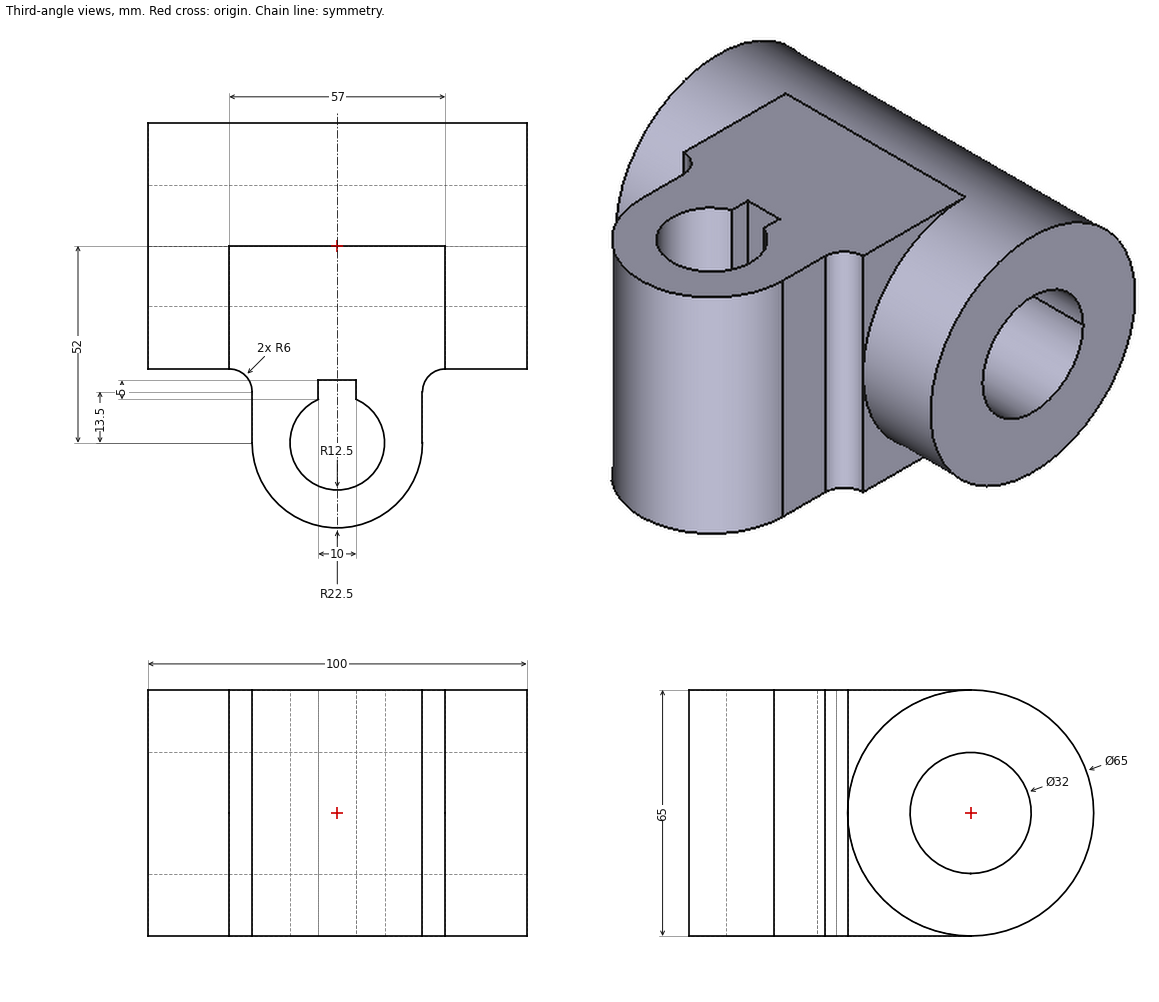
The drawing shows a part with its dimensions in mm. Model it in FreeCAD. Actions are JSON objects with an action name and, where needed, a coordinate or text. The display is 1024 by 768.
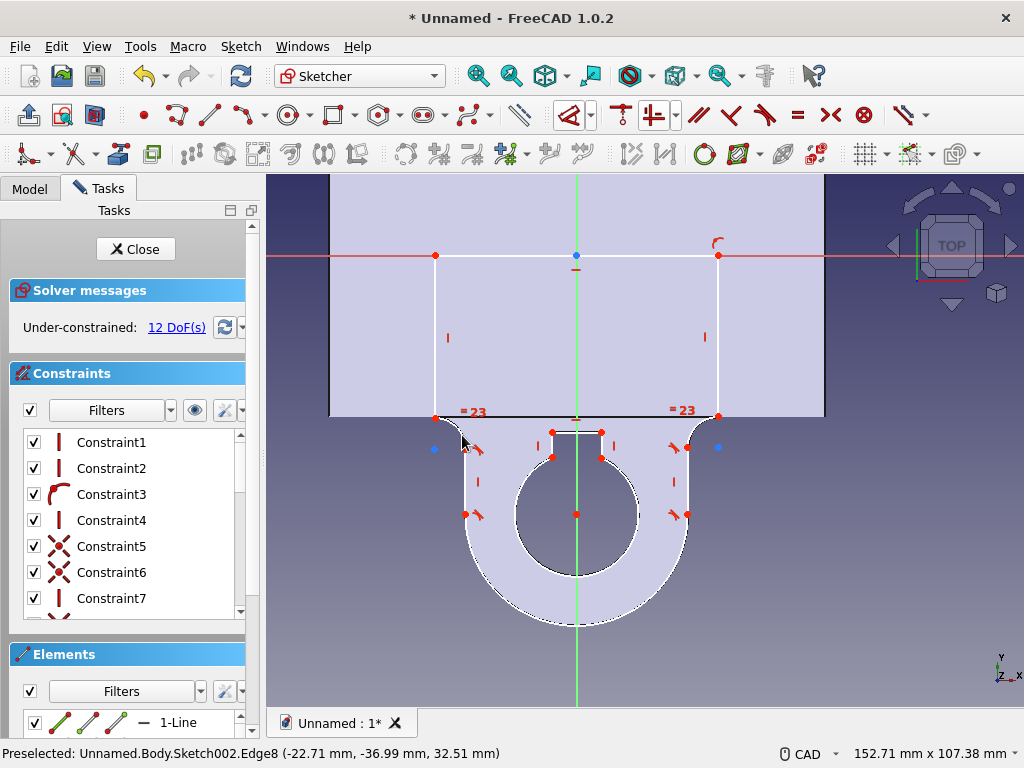
{"action": "left_click", "coordinate": [576, 515]}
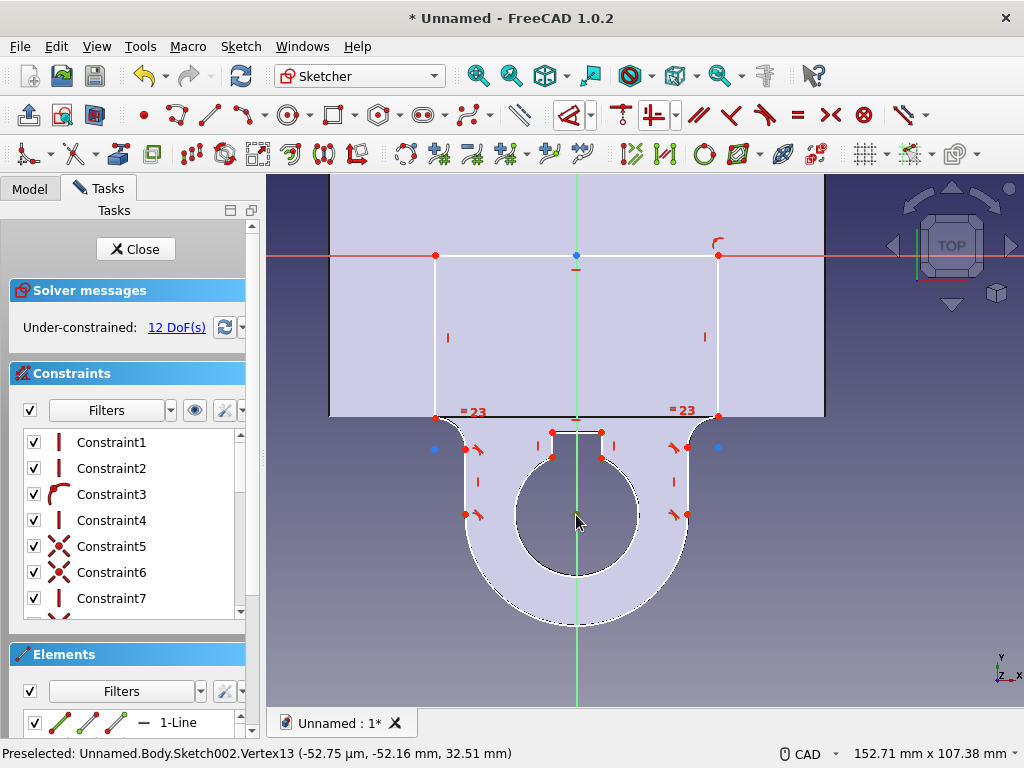
{"action": "left_click", "coordinate": [577, 543]}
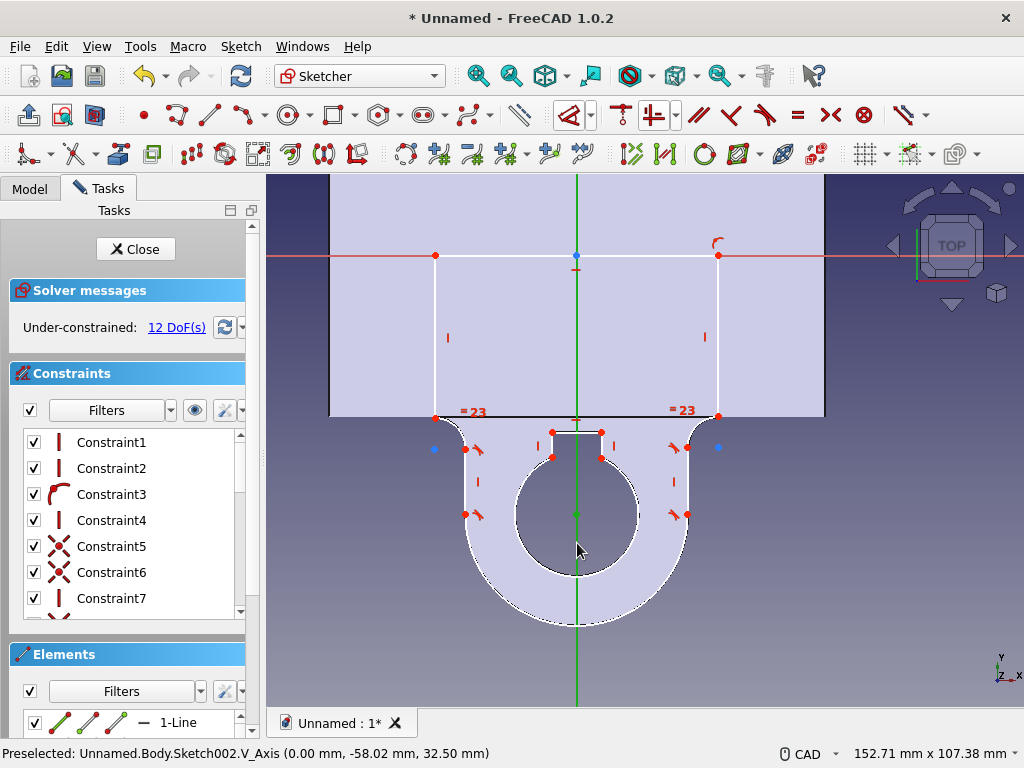
{"action": "key", "text": "c"}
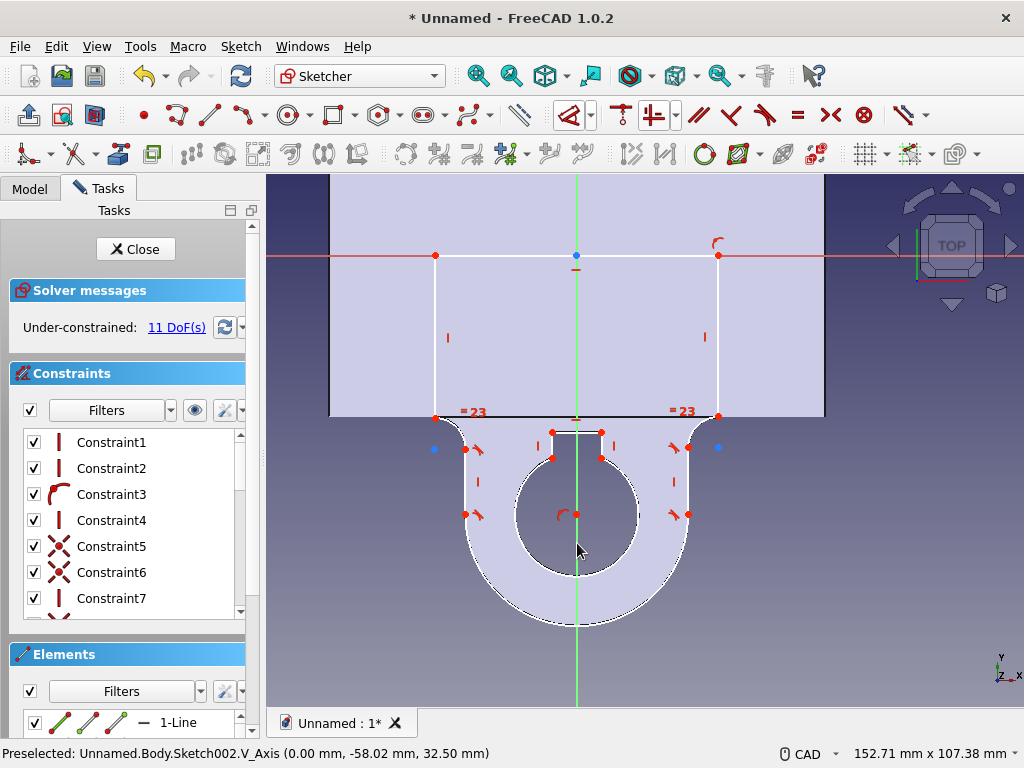
{"action": "left_click", "coordinate": [718, 417]}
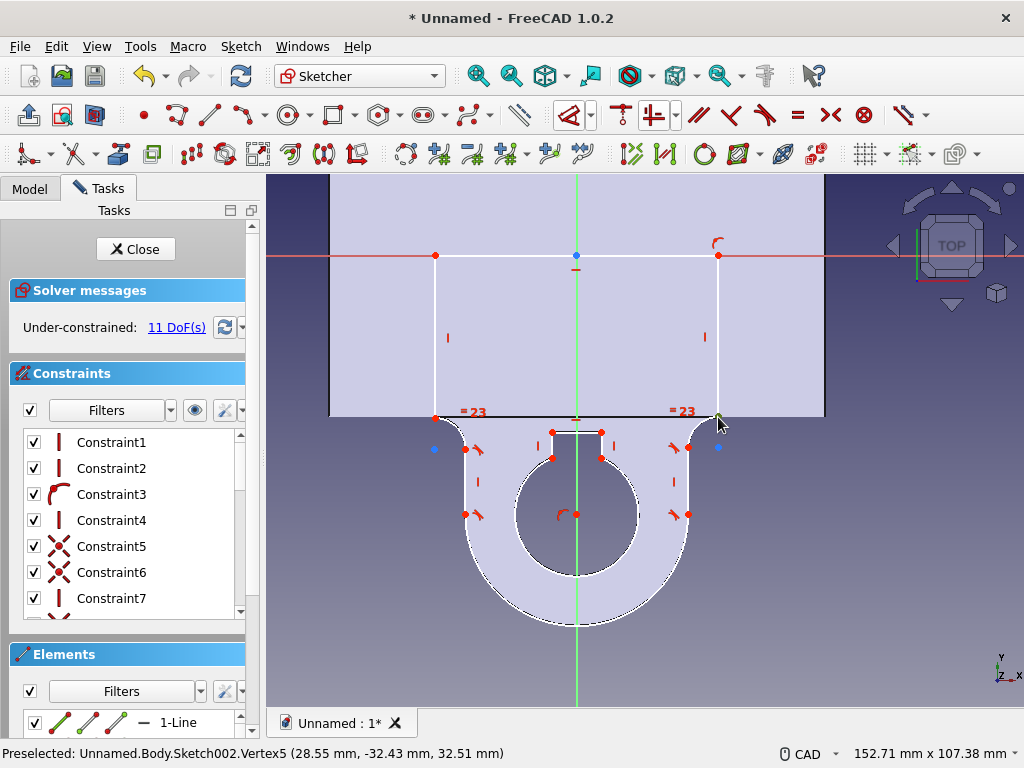
{"action": "left_click", "coordinate": [435, 418]}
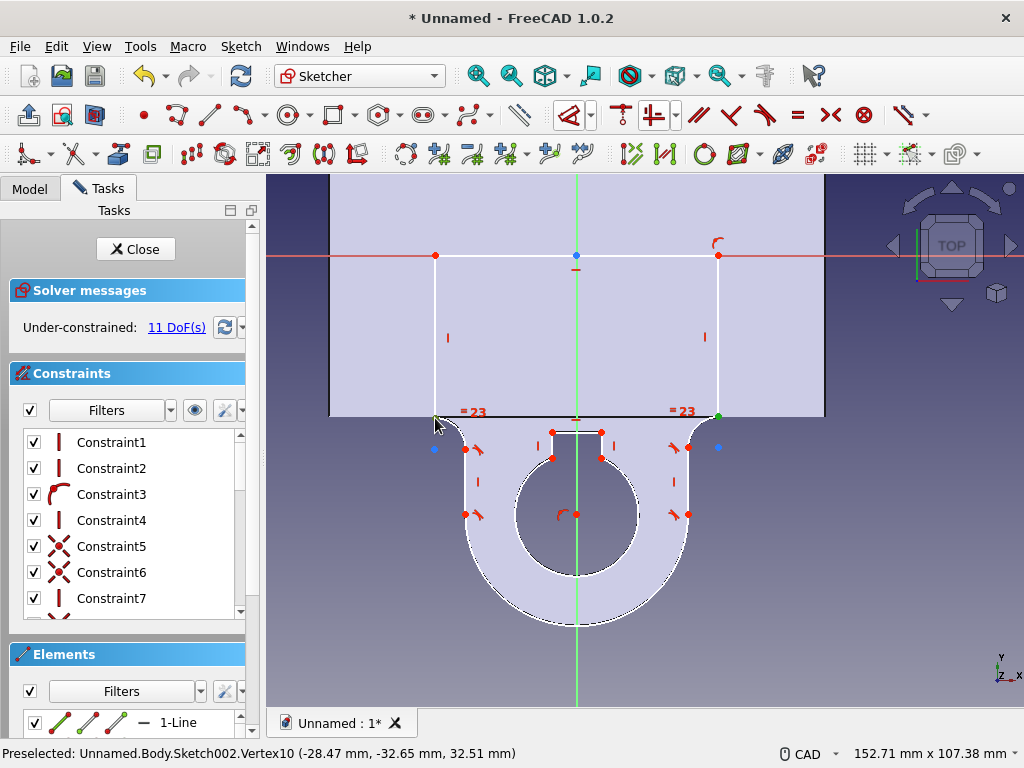
{"action": "left_click", "coordinate": [577, 543]}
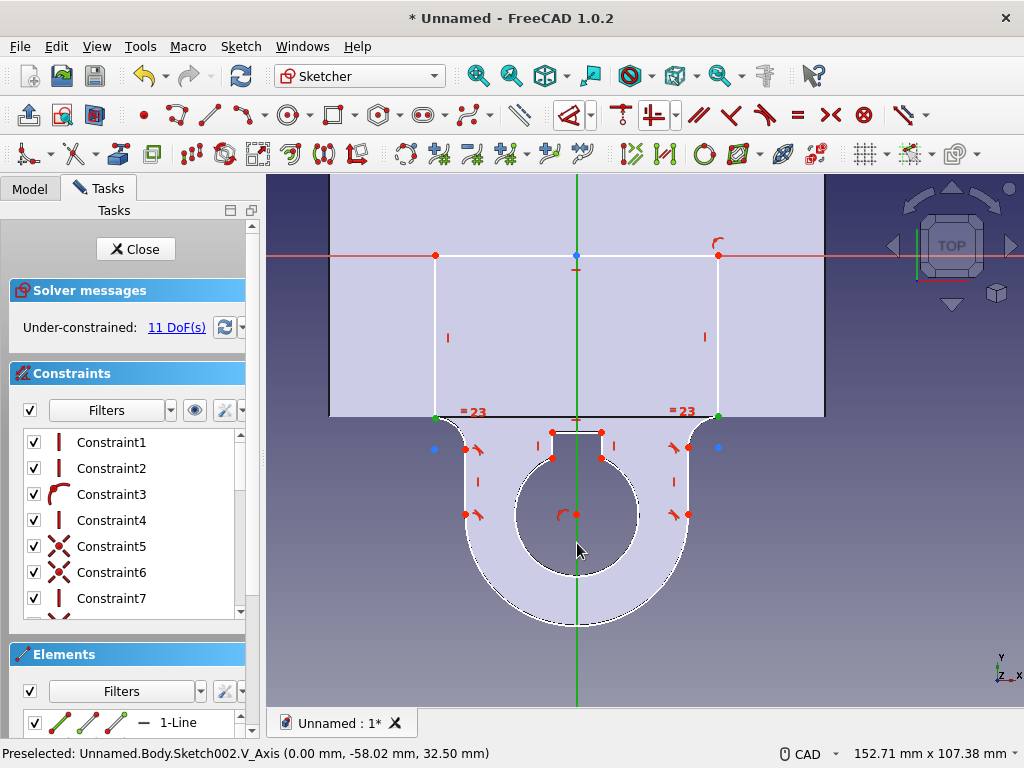
{"action": "left_click", "coordinate": [831, 116]}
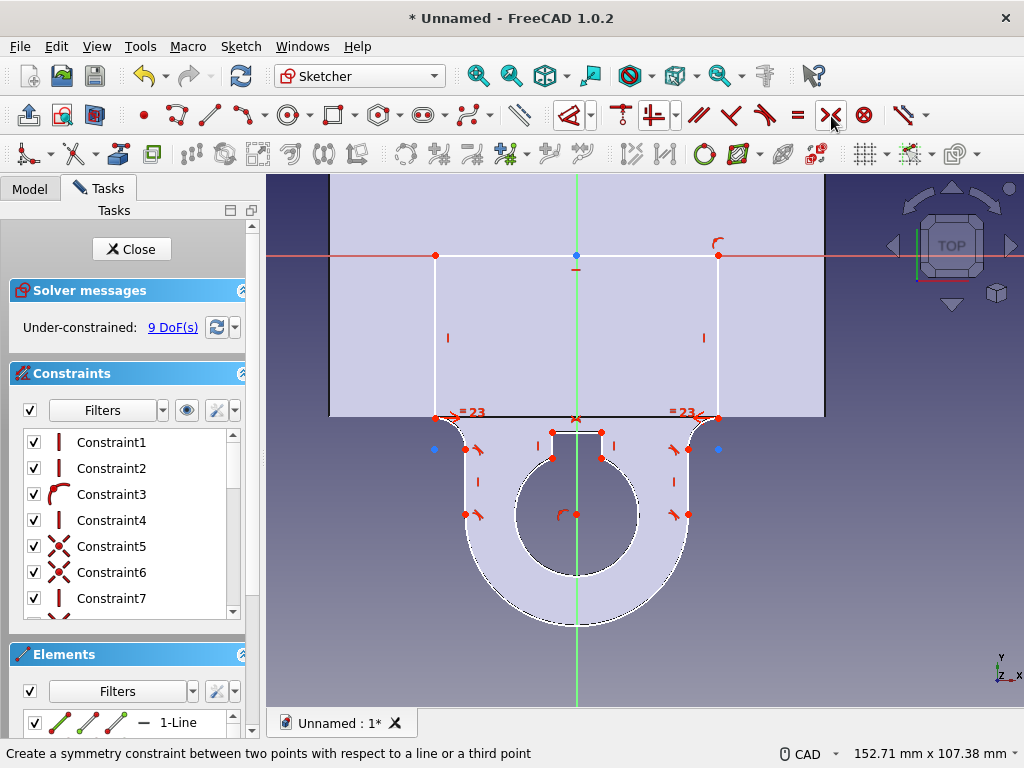
{"action": "left_click", "coordinate": [511, 605]}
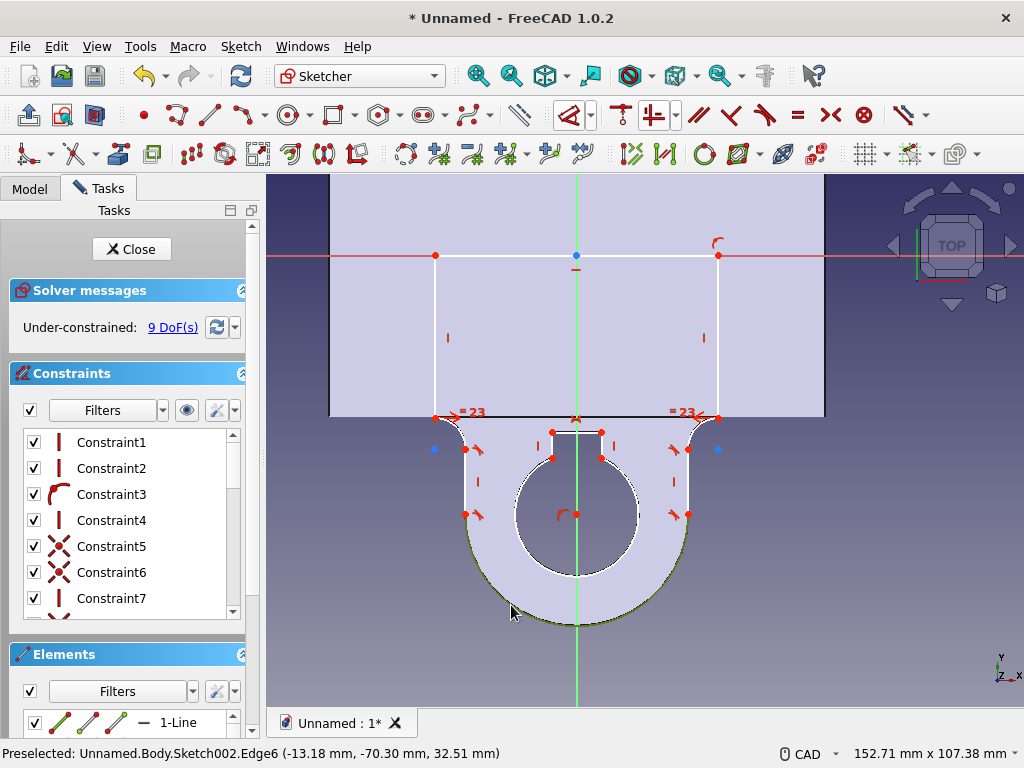
{"action": "key", "text": "k r"}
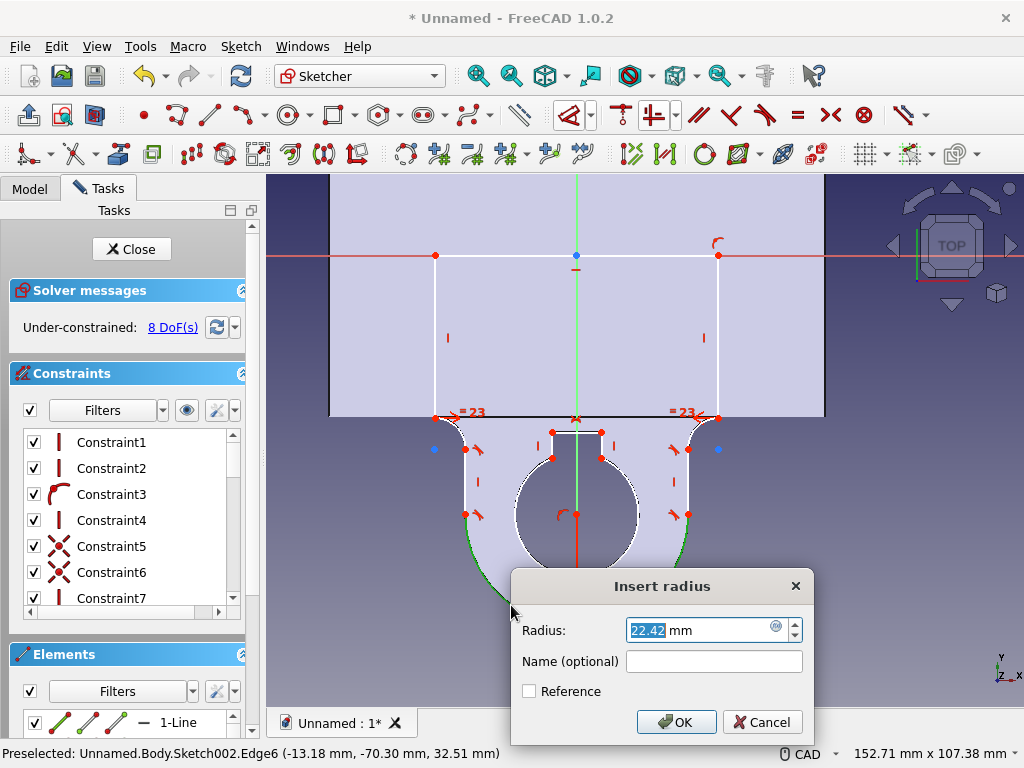
{"action": "type", "text": "22.5"}
{"action": "key", "text": "Return"}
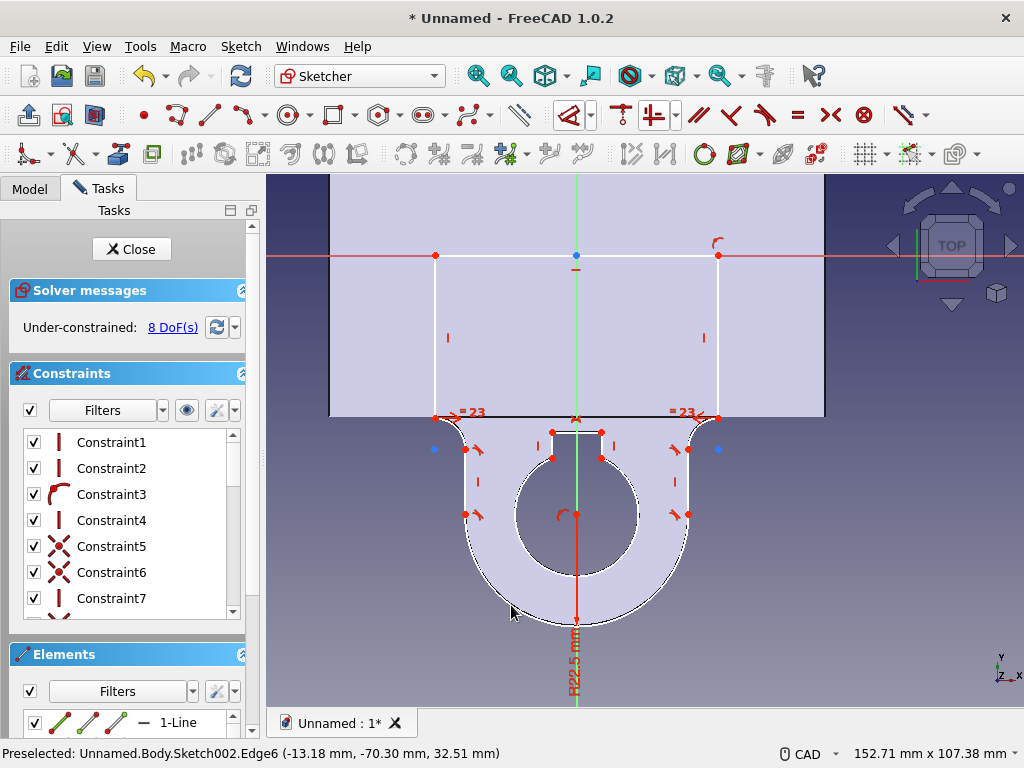
{"action": "scroll", "coordinate": [705, 422], "scroll_direction": "up", "scroll_amount": 2}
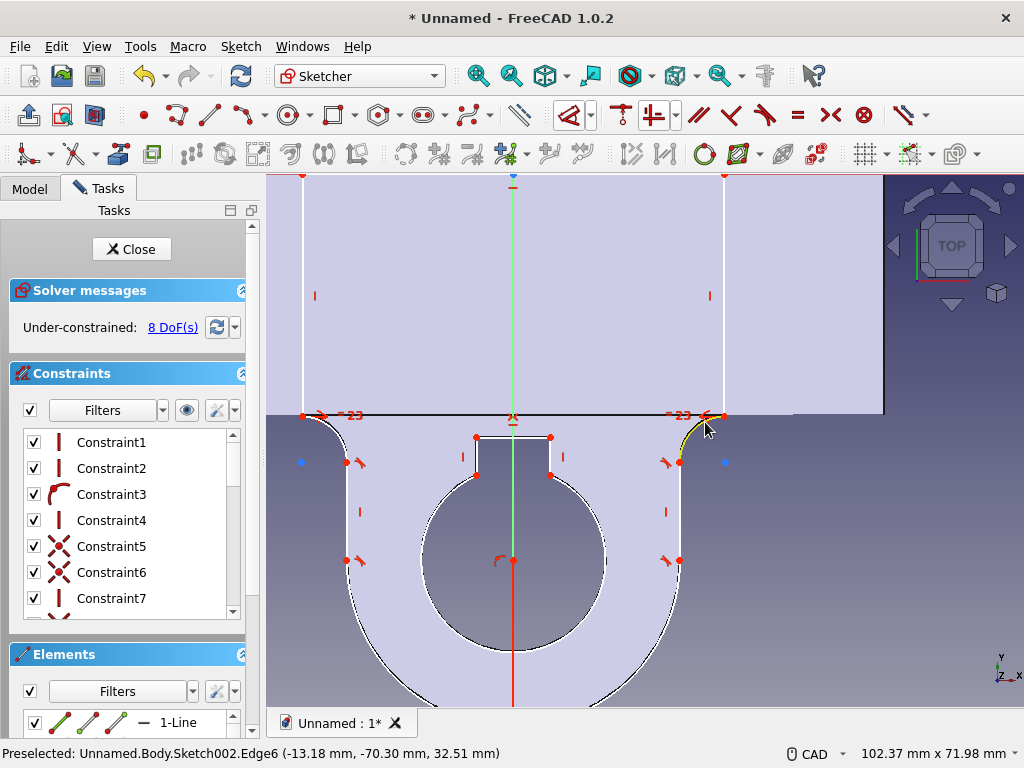
{"action": "left_click", "coordinate": [704, 422]}